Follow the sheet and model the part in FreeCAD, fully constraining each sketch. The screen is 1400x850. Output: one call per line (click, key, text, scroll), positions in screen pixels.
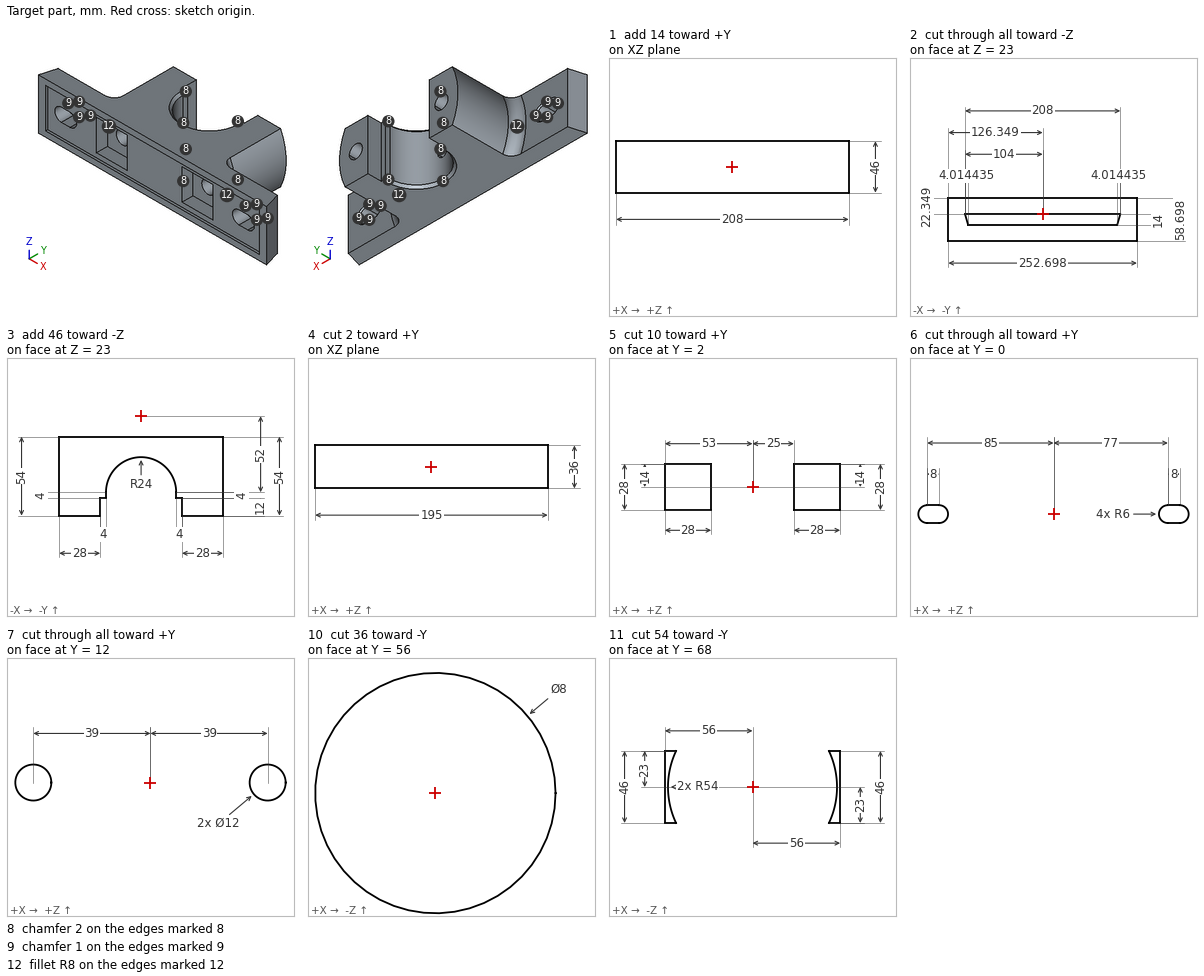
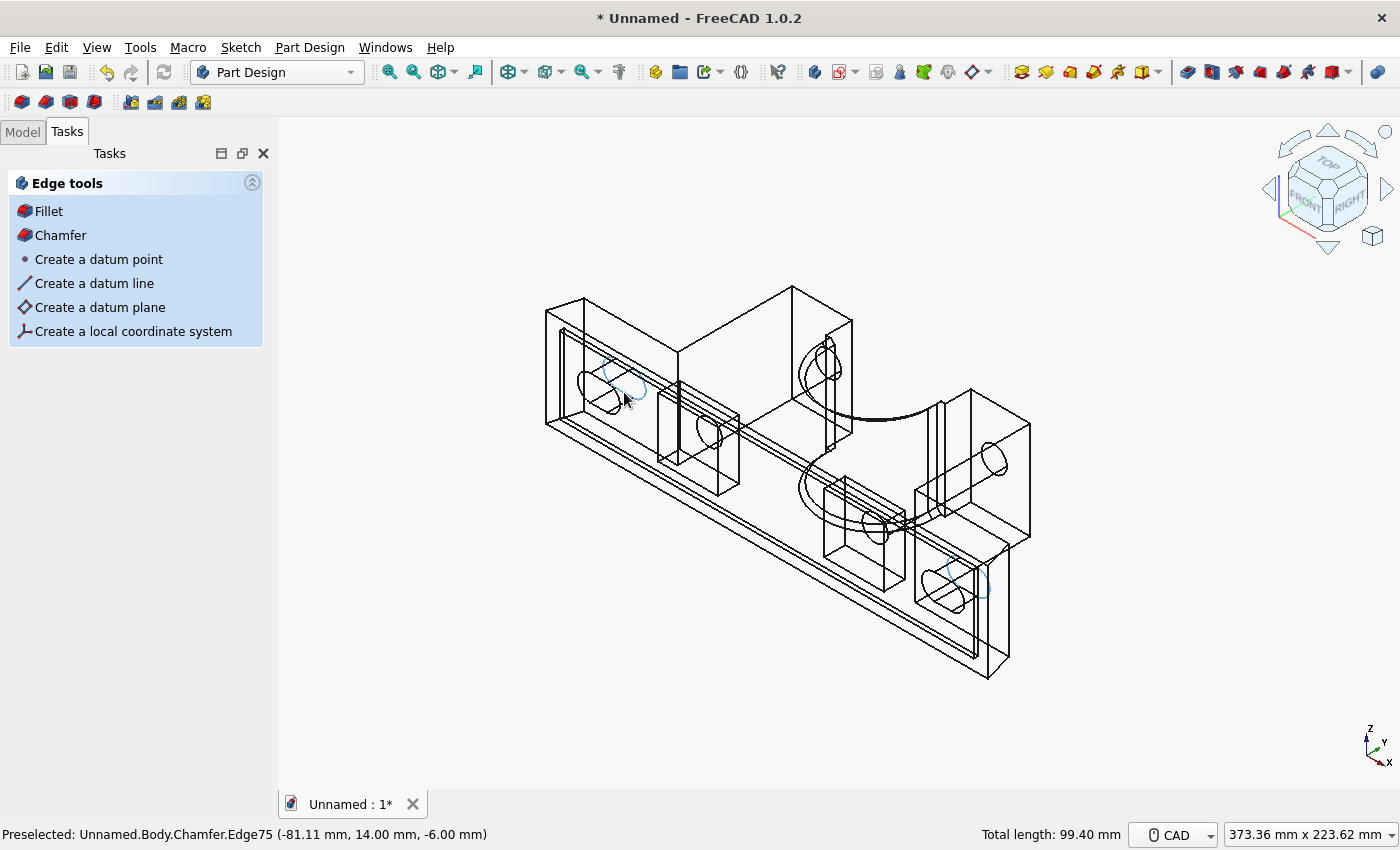
key(2)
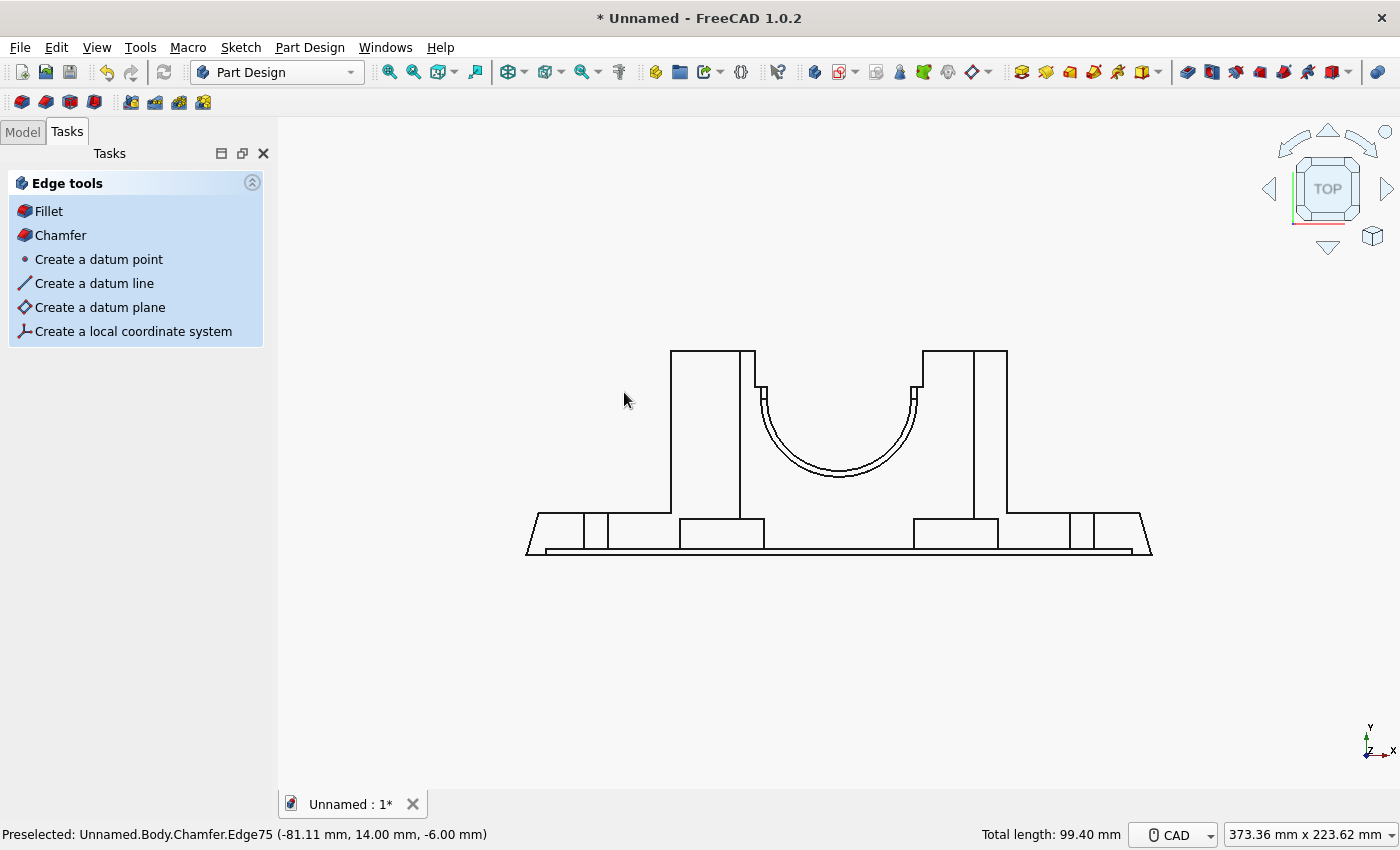
key(1)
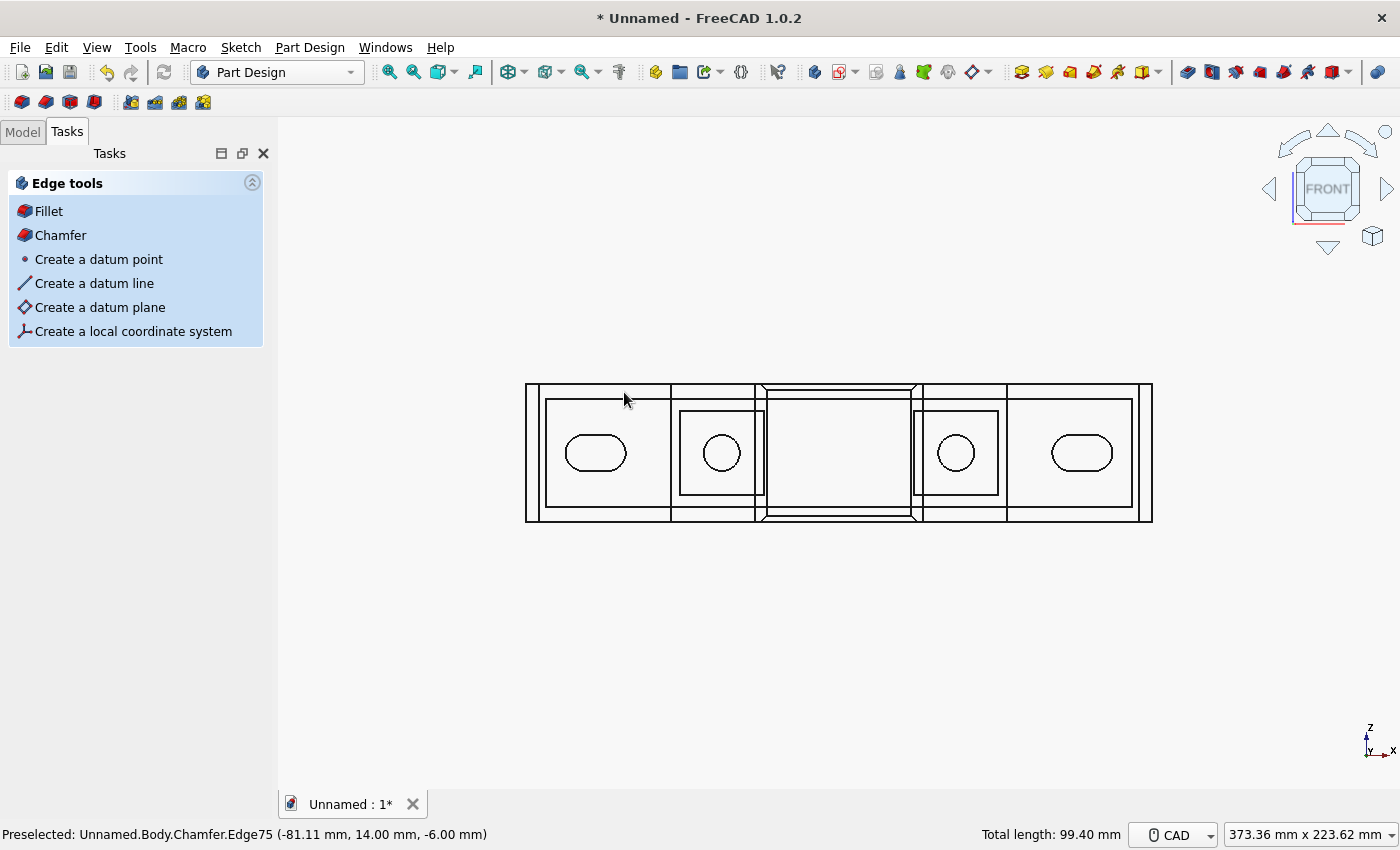
key(3)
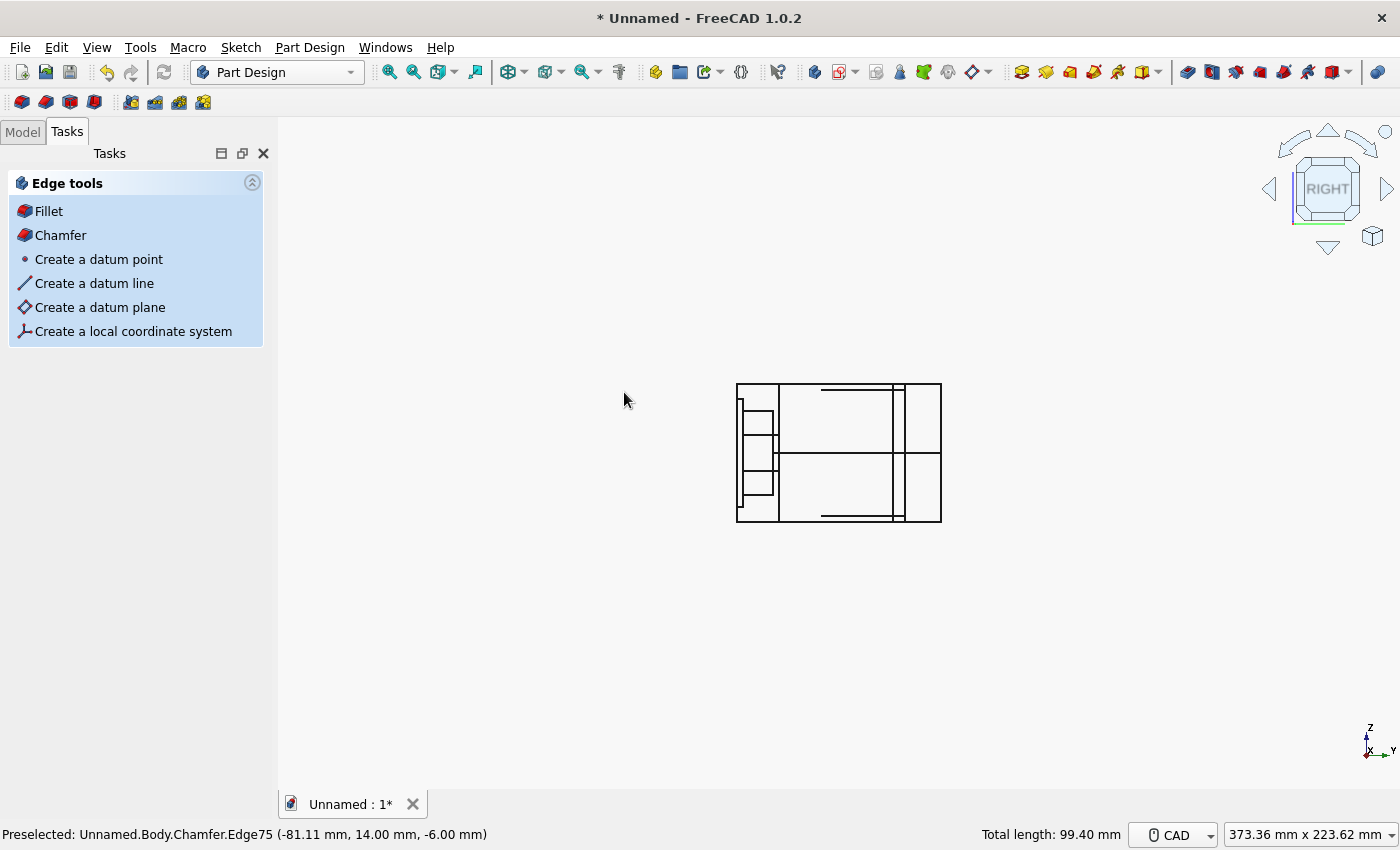
key(v)
key(f)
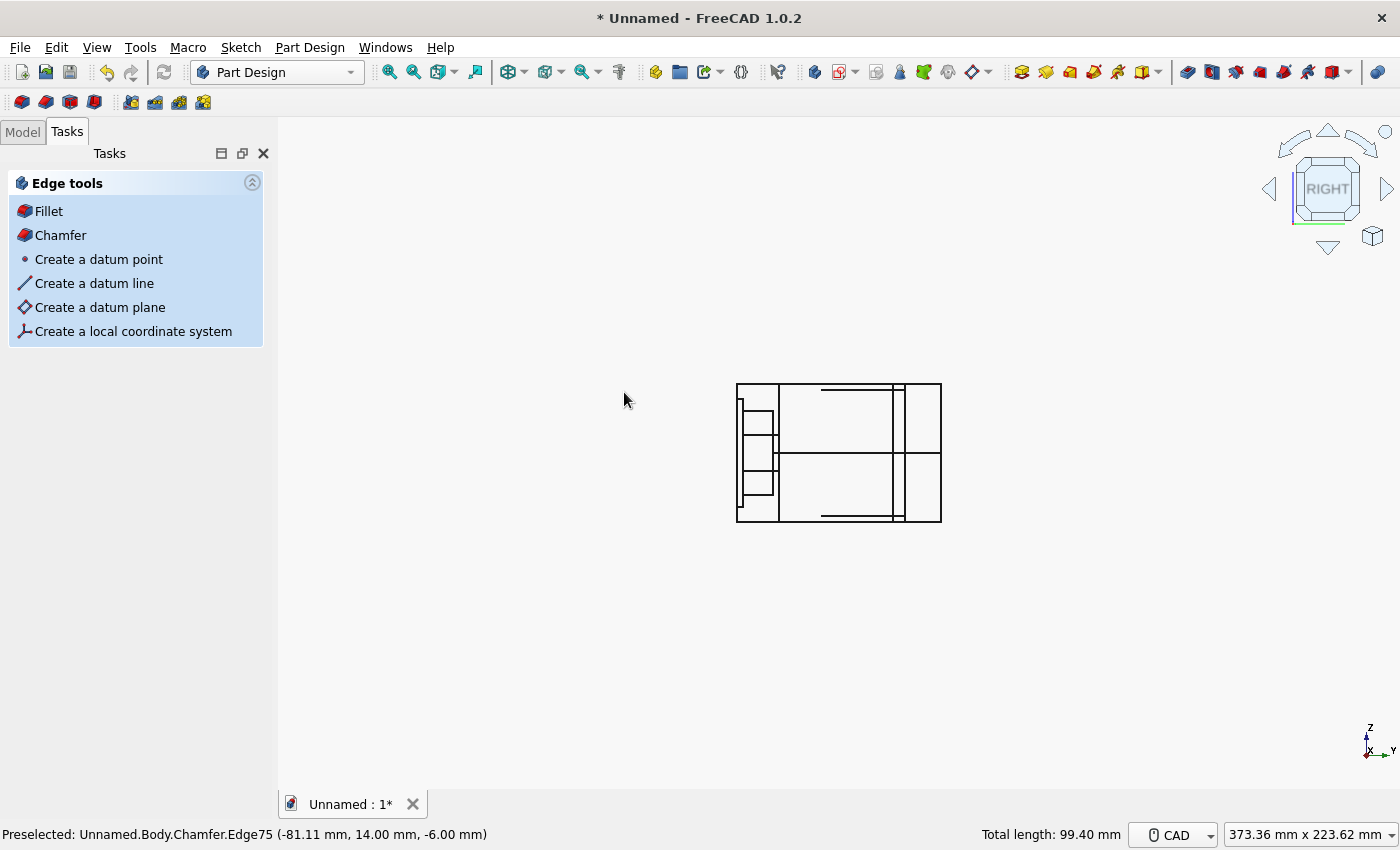
key(5)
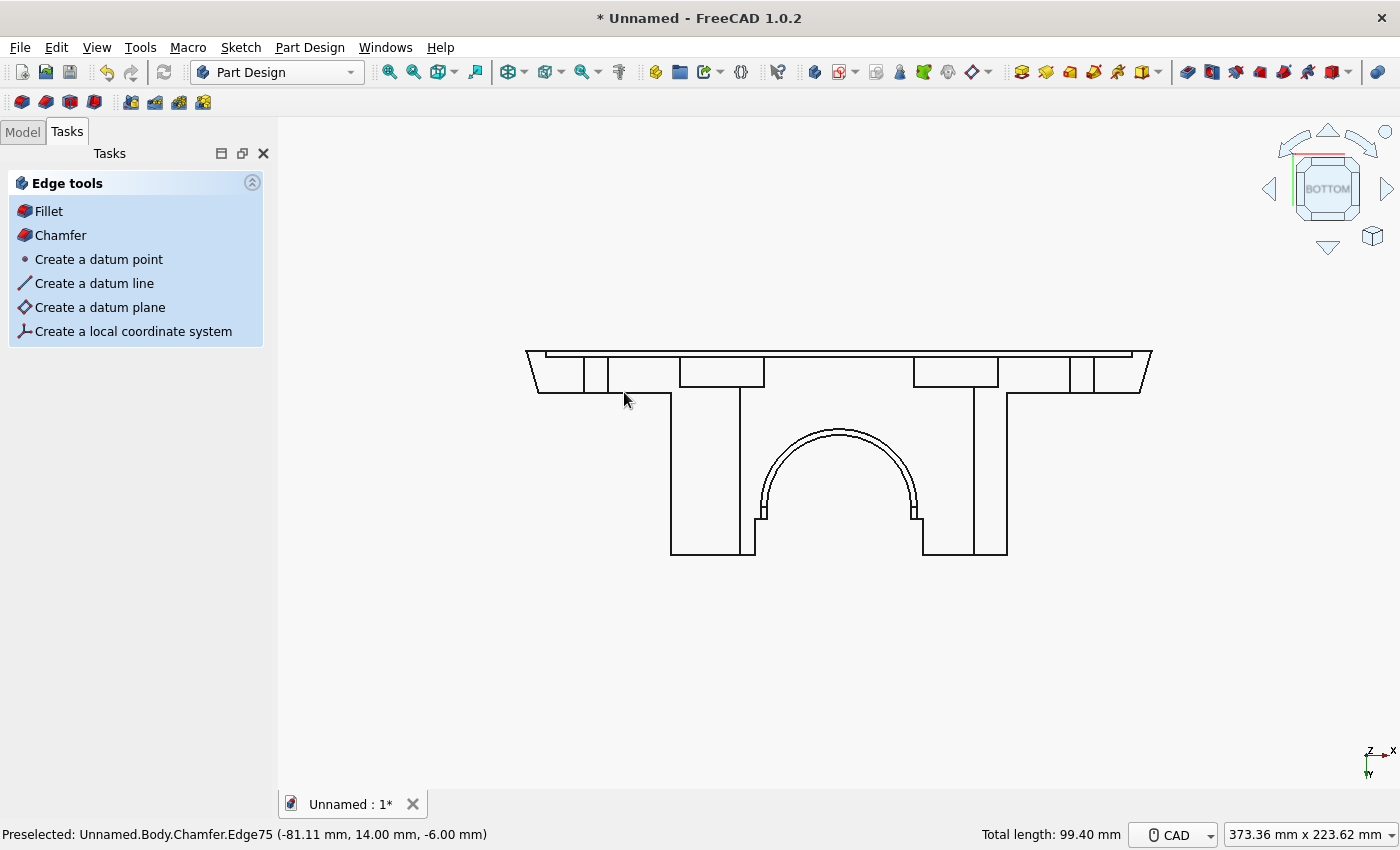
key(4)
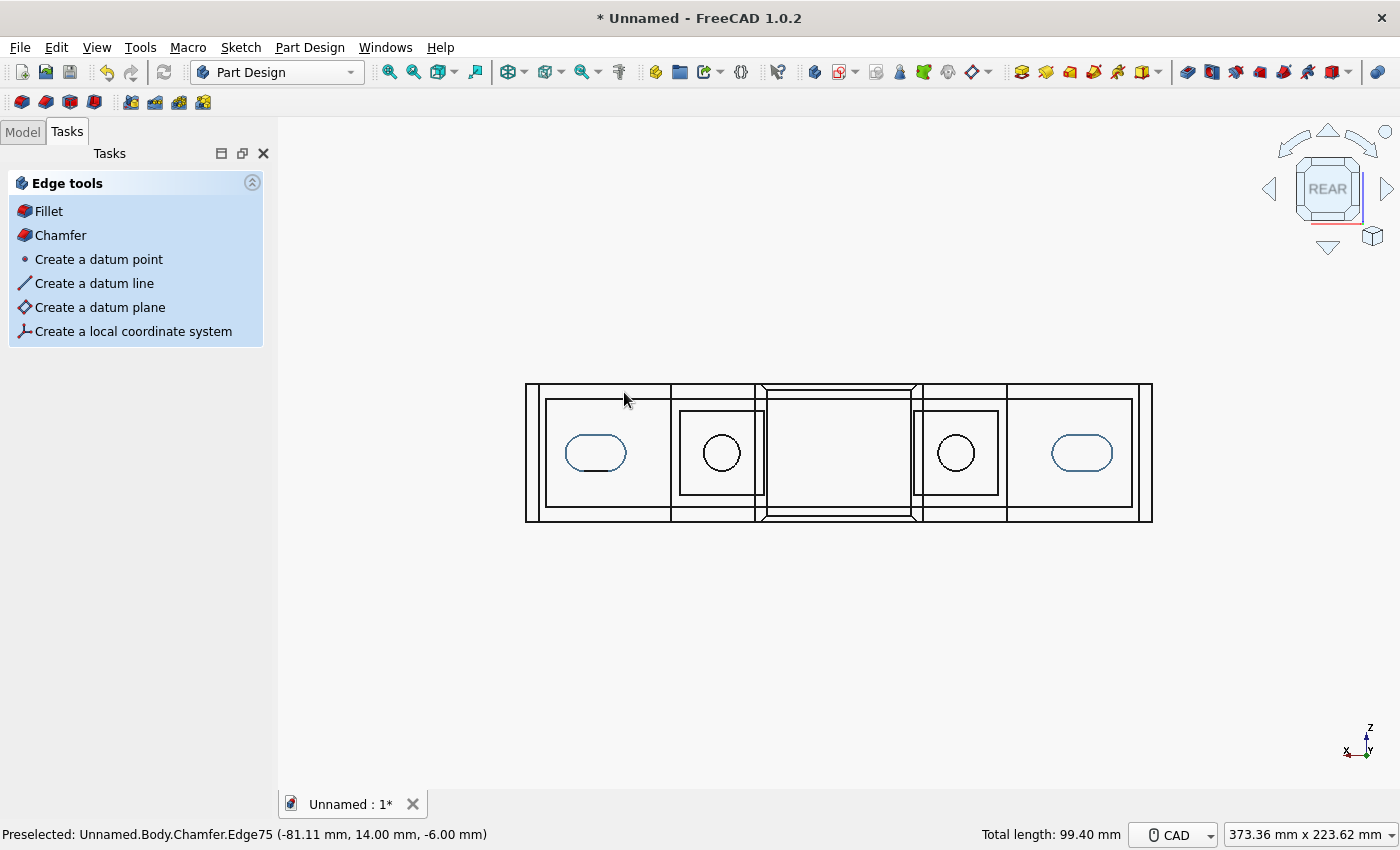
click(596, 470, ctrl)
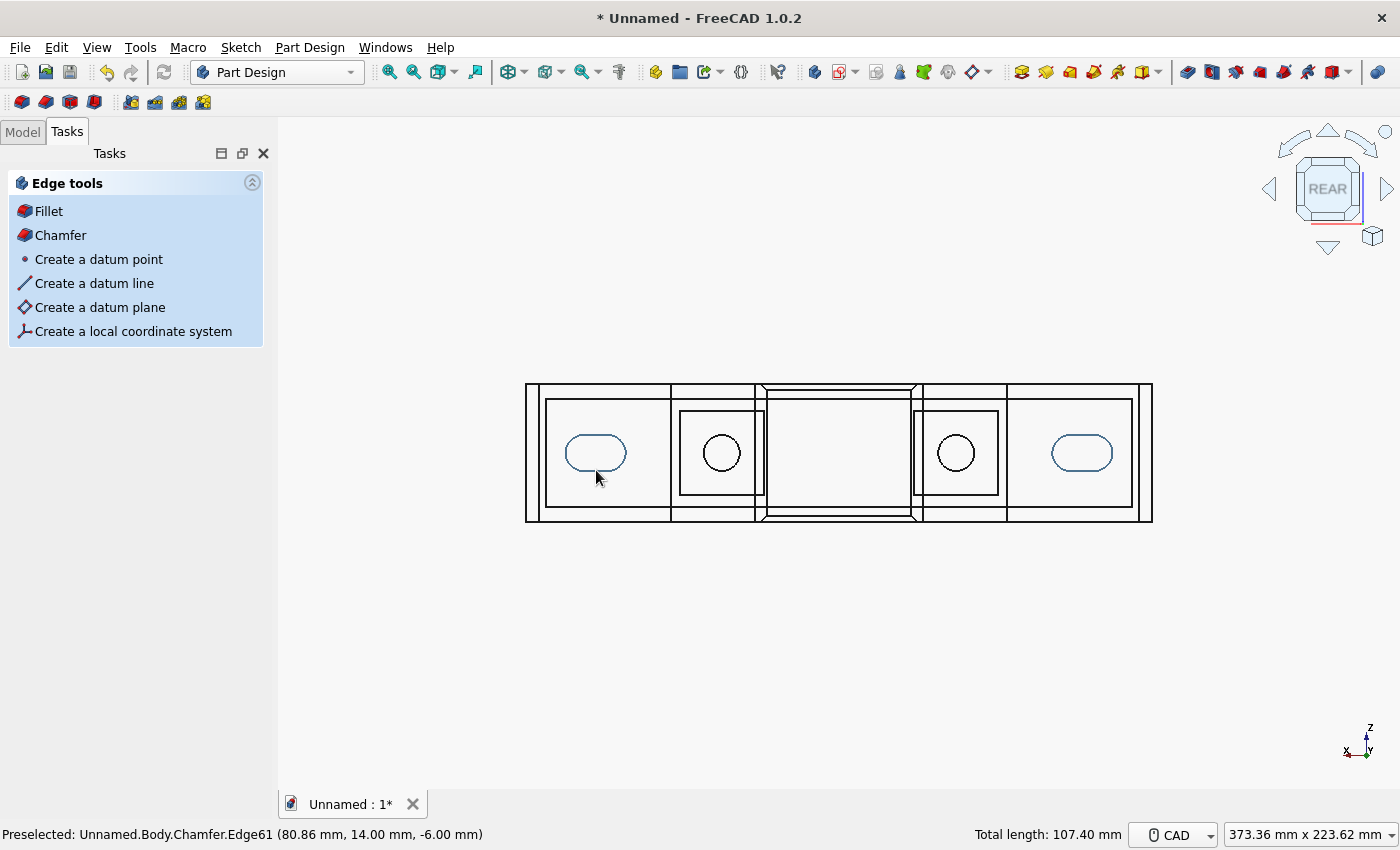
key(v)
key(1)